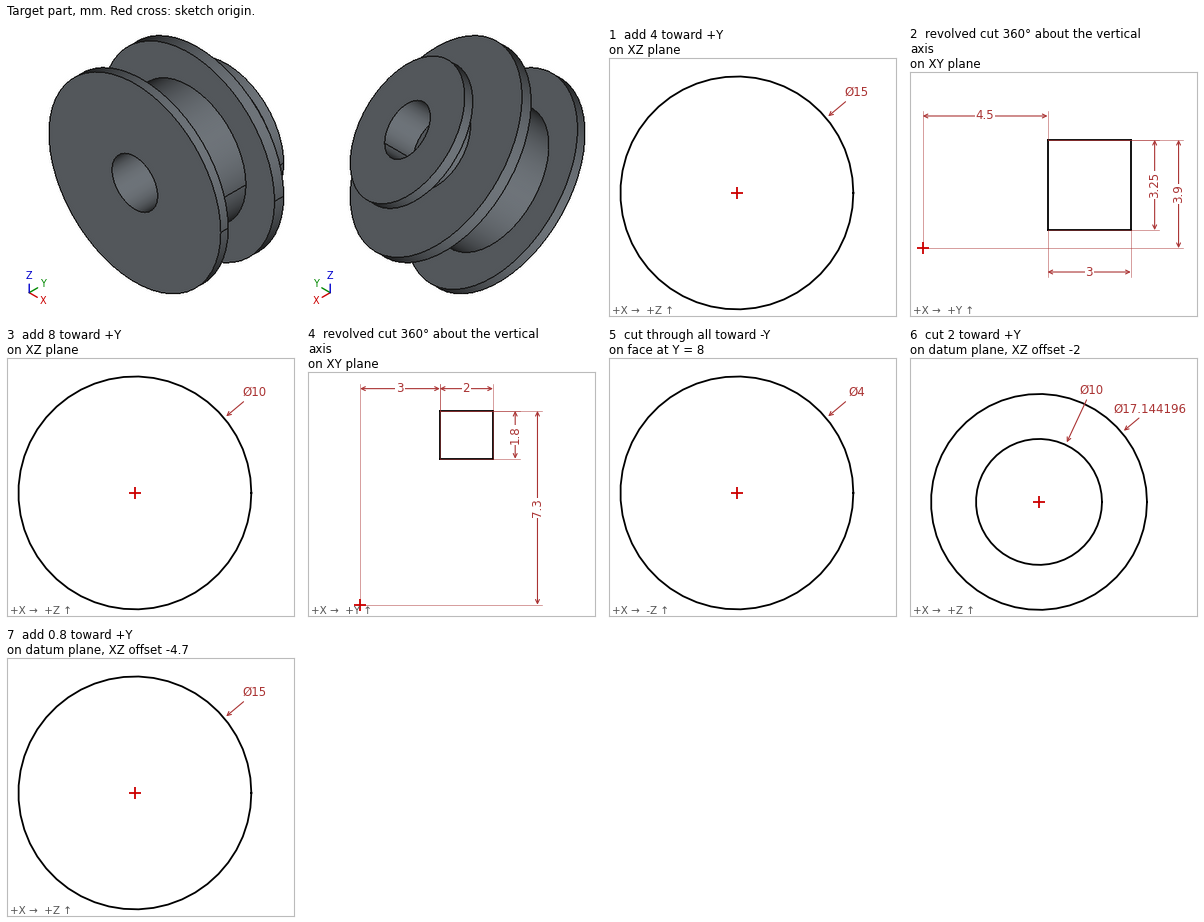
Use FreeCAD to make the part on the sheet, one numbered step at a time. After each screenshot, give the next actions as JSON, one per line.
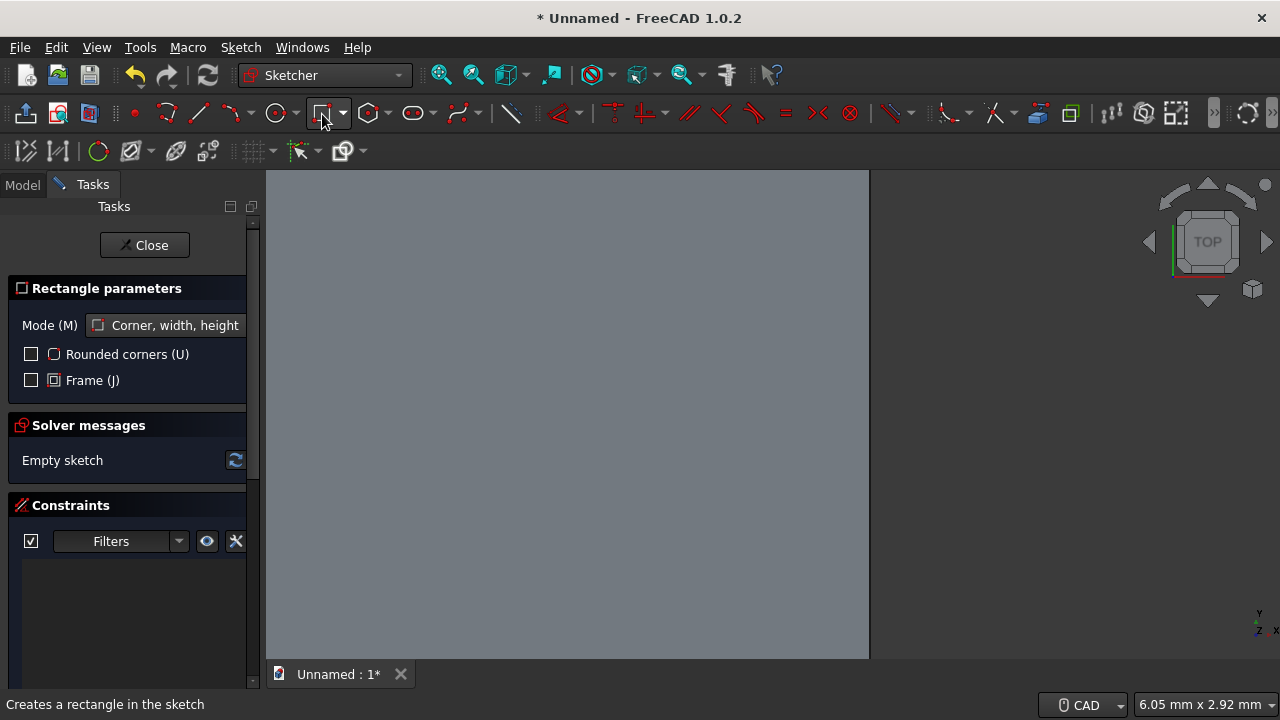
{"action": "left_click", "coordinate": [535, 259]}
{"action": "left_click", "coordinate": [870, 561]}
{"action": "key", "text": "Escape"}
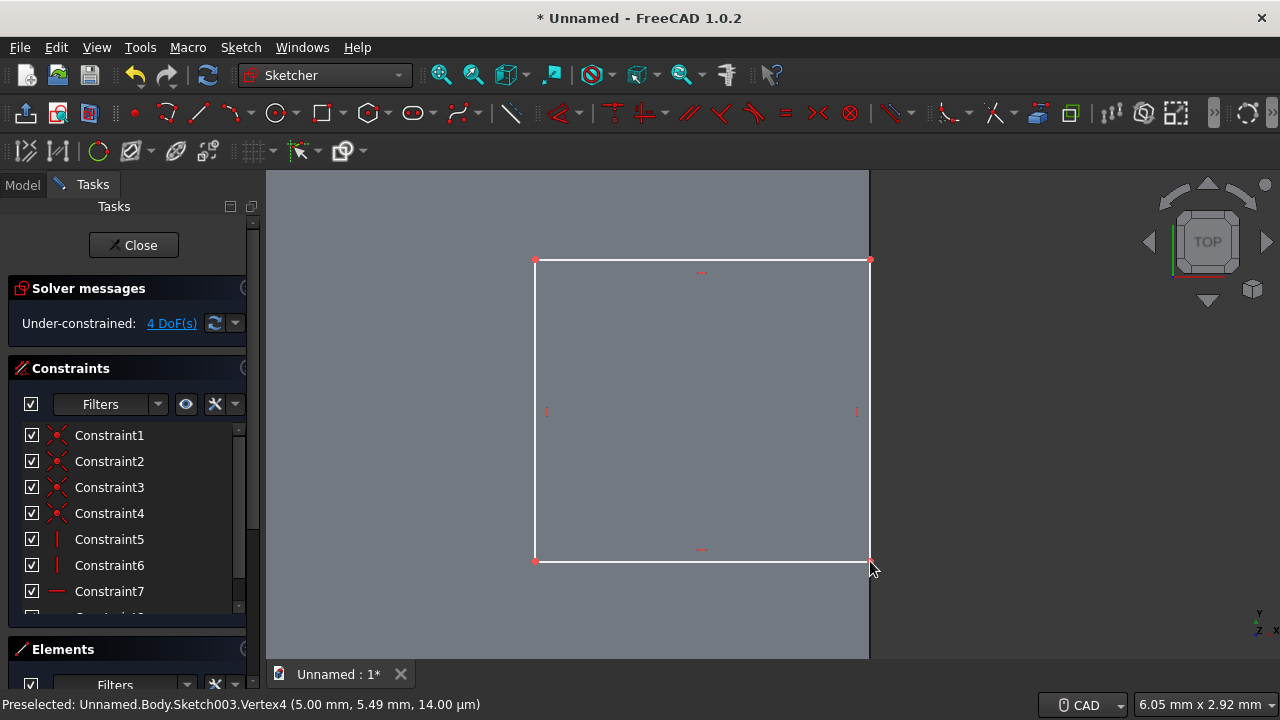
{"action": "left_click", "coordinate": [558, 114]}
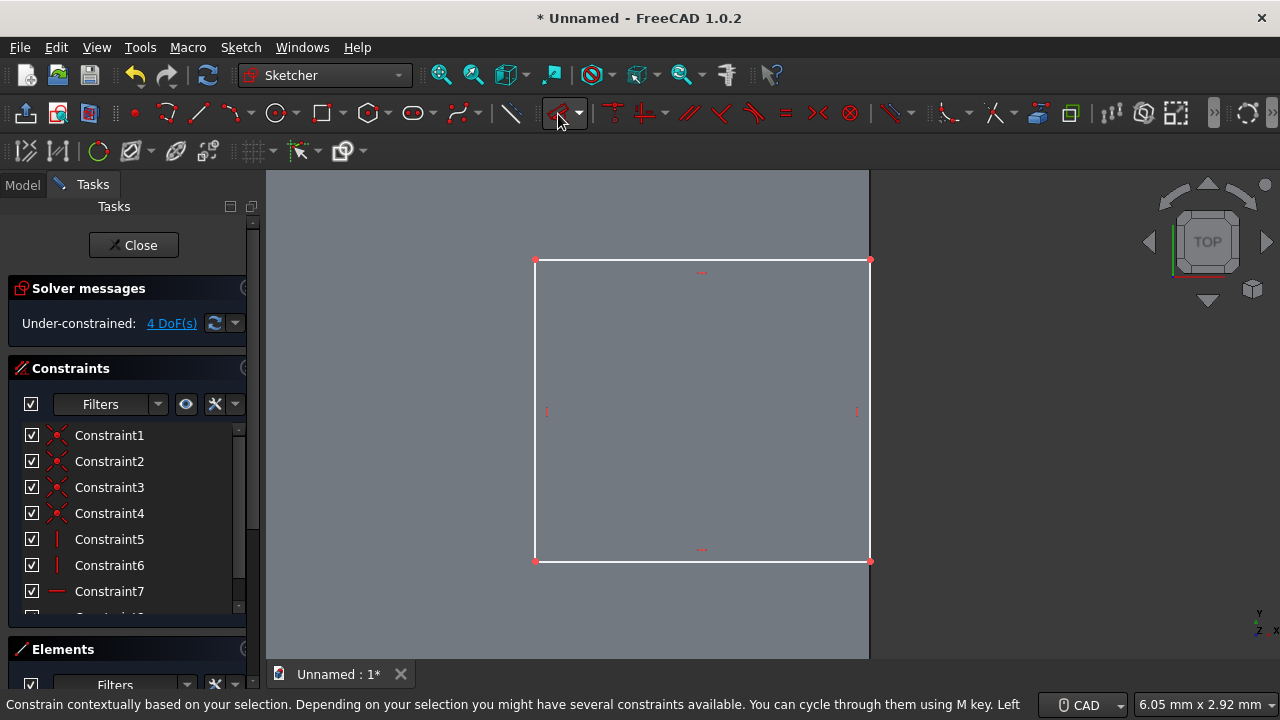
{"action": "left_click", "coordinate": [636, 562]}
{"action": "left_click", "coordinate": [703, 596]}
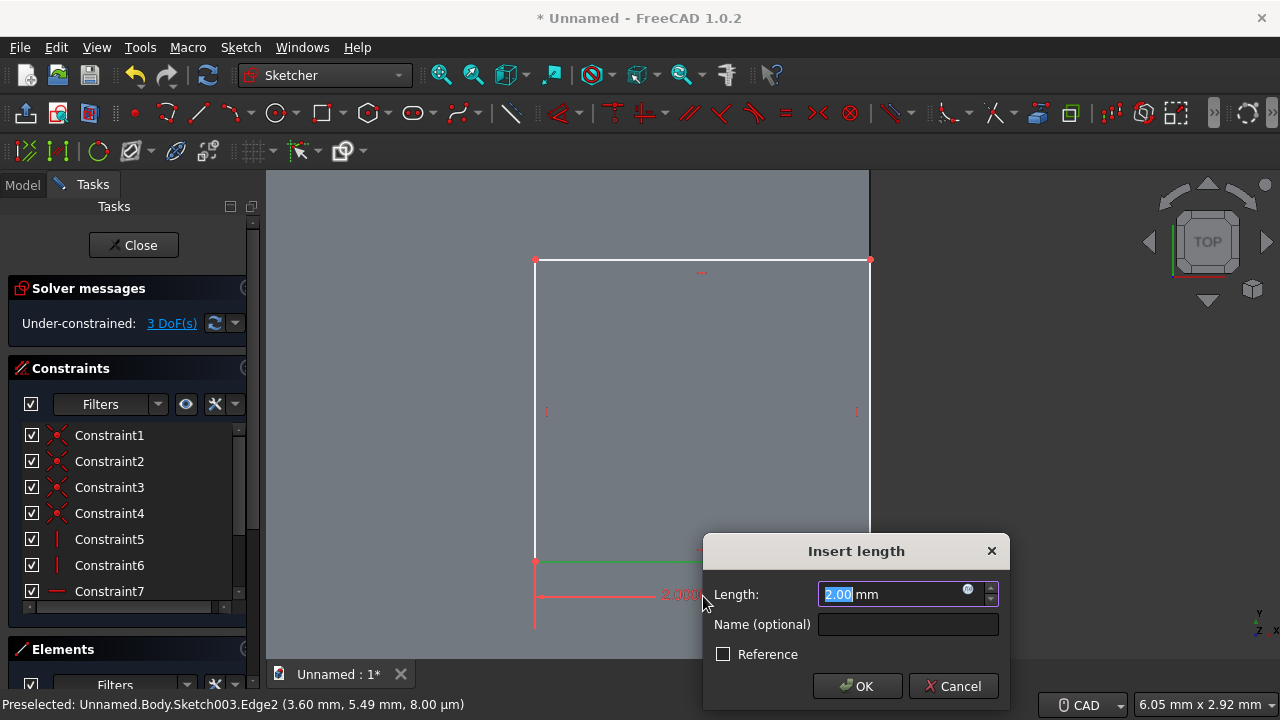
{"action": "type", "text": "2"}
{"action": "key", "text": "Return"}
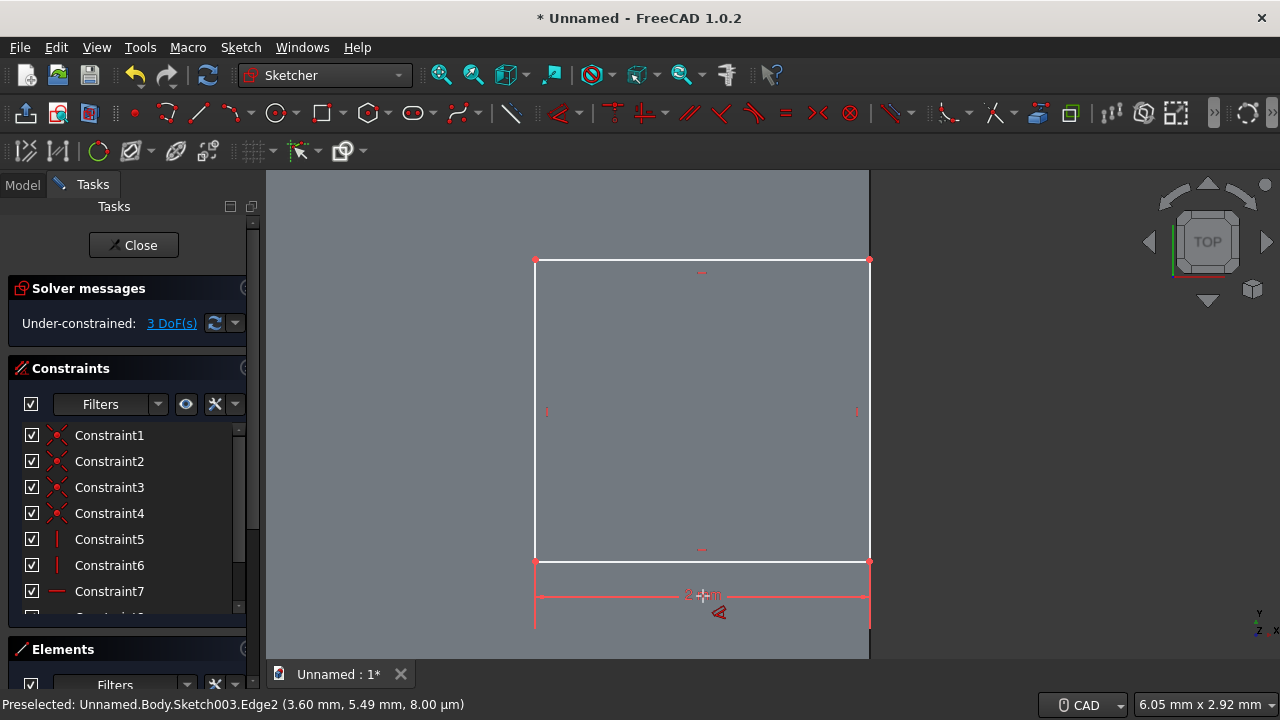
{"action": "left_click", "coordinate": [535, 260]}
{"action": "left_click", "coordinate": [415, 226]}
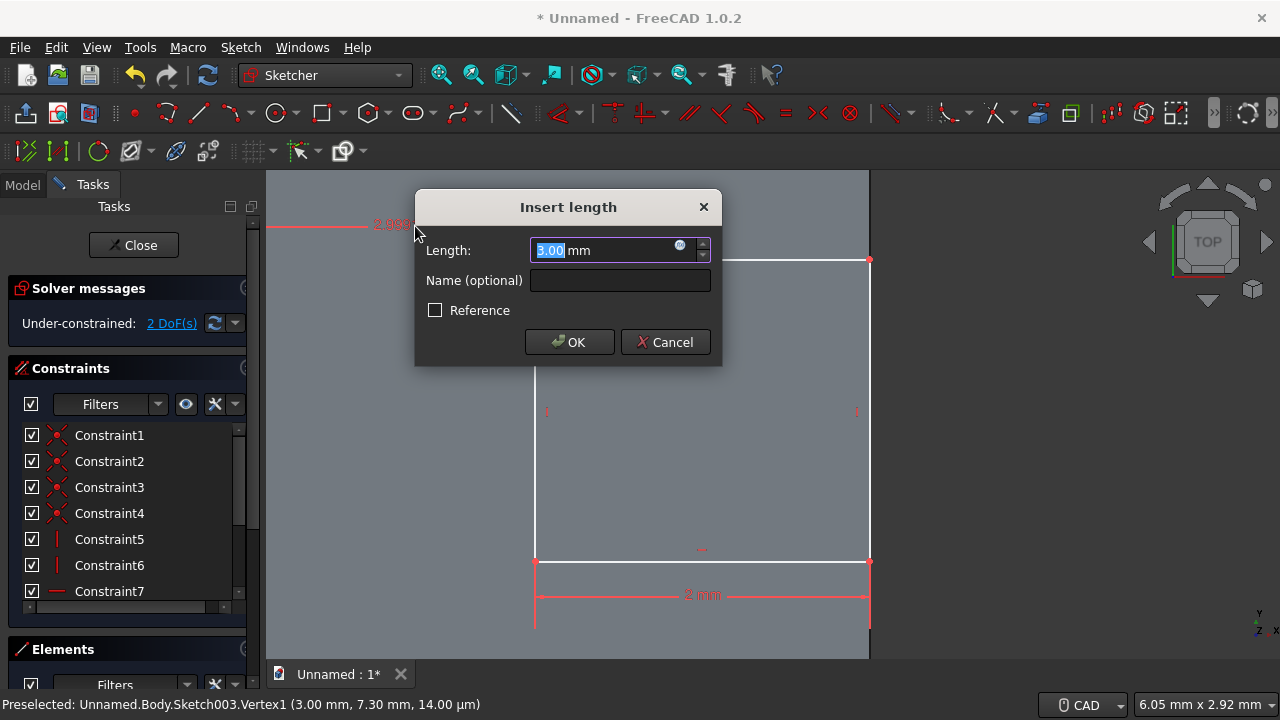
{"action": "type", "text": "3"}
{"action": "key", "text": "Return"}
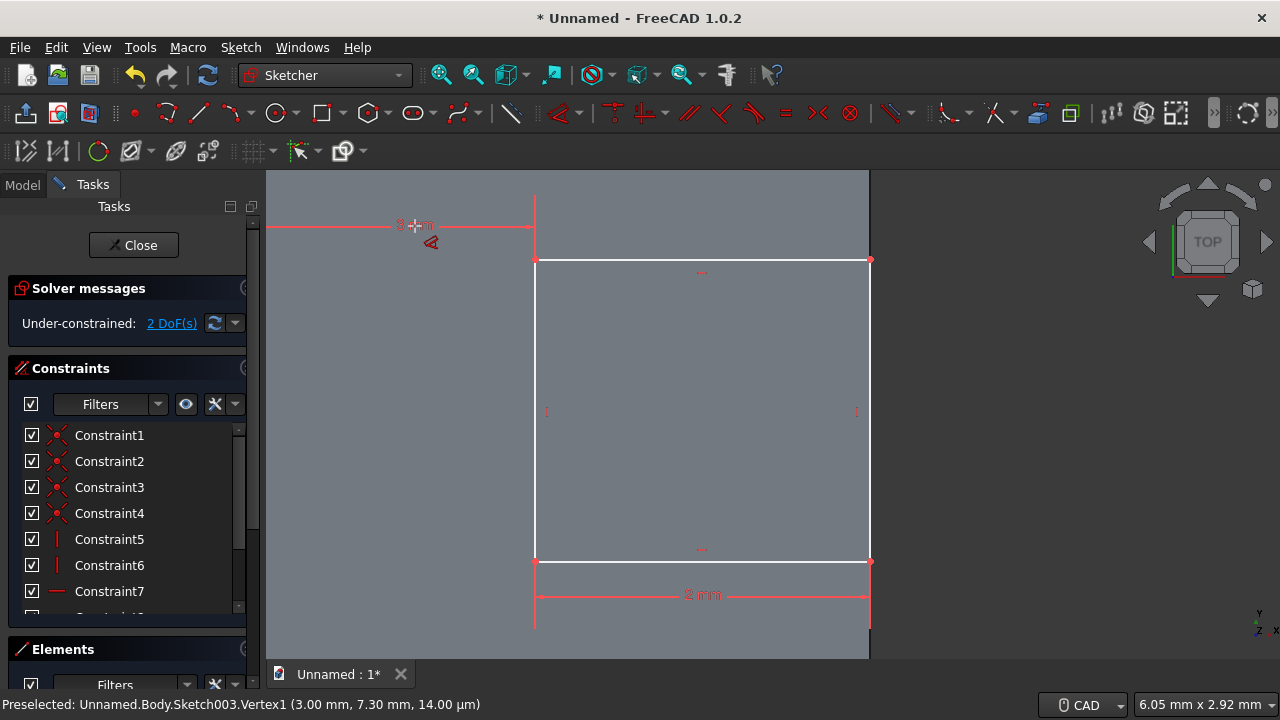
{"action": "left_click", "coordinate": [535, 351]}
{"action": "left_click", "coordinate": [501, 411]}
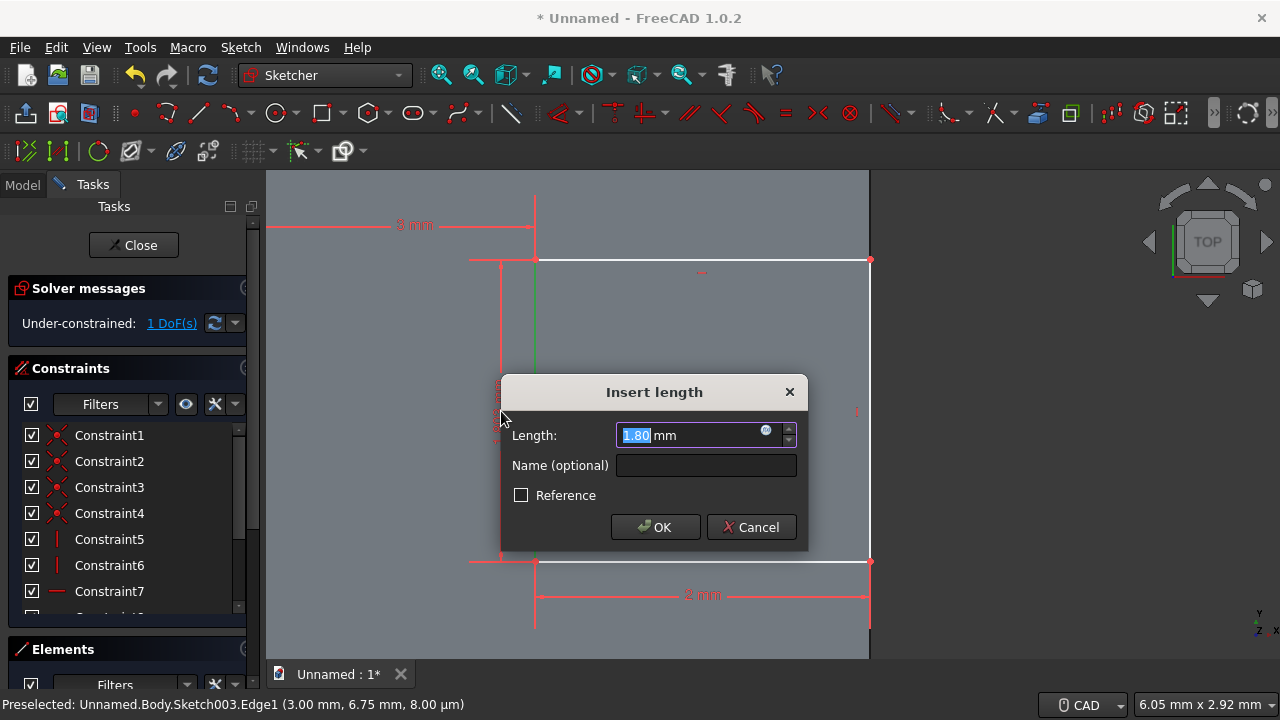
{"action": "type", "text": "1.8"}
{"action": "key", "text": "Return"}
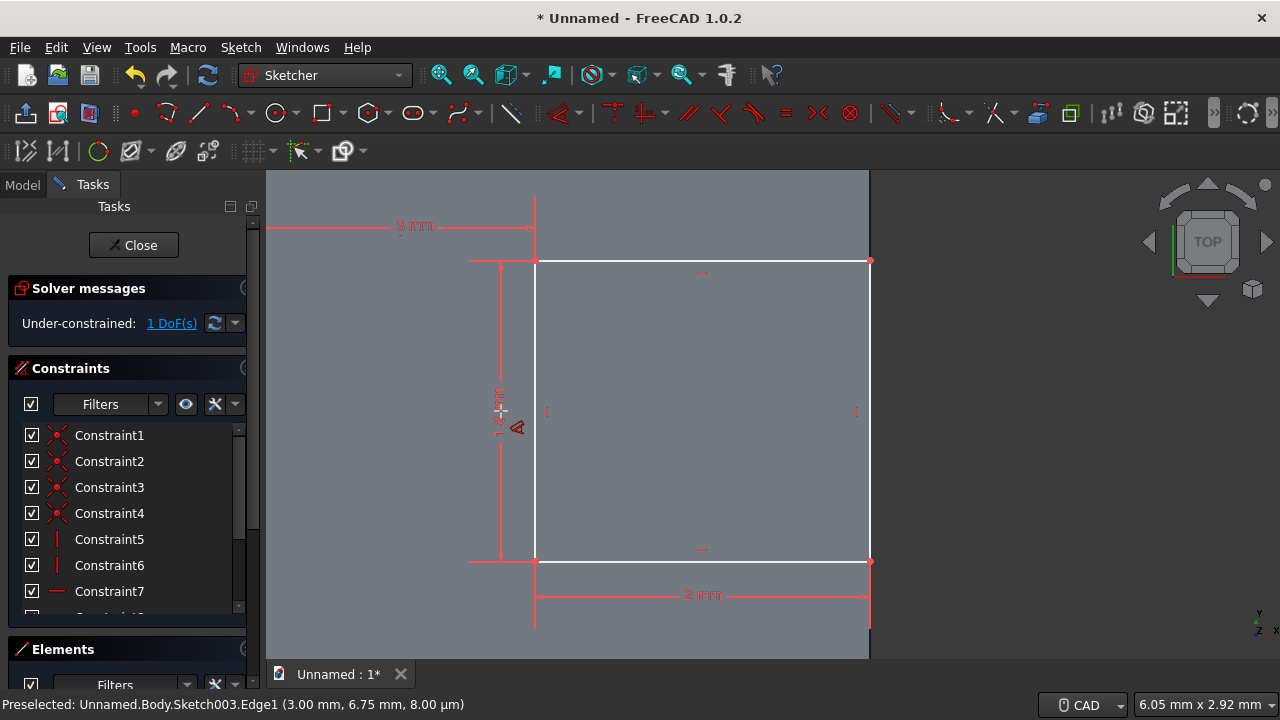
{"action": "left_click", "coordinate": [535, 261]}
{"action": "left_click", "coordinate": [569, 446]}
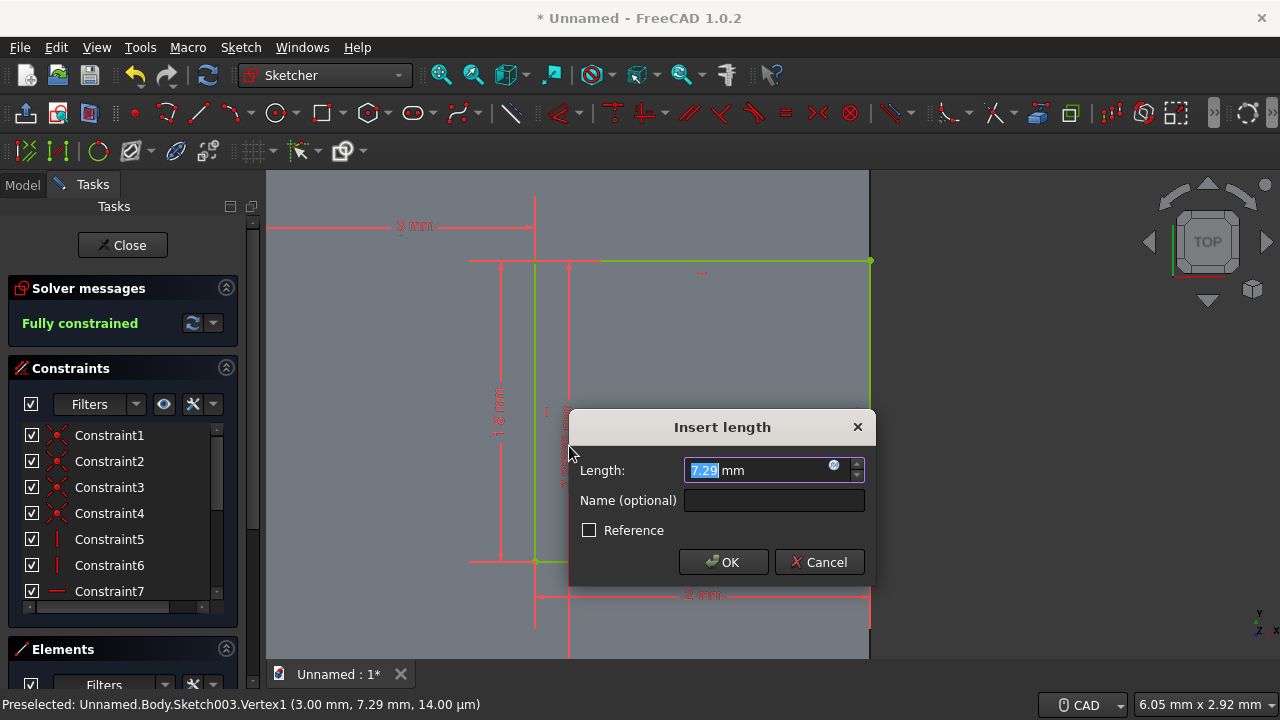
{"action": "type", "text": "7.3"}
{"action": "key", "text": "Return"}
{"action": "key", "text": "Escape"}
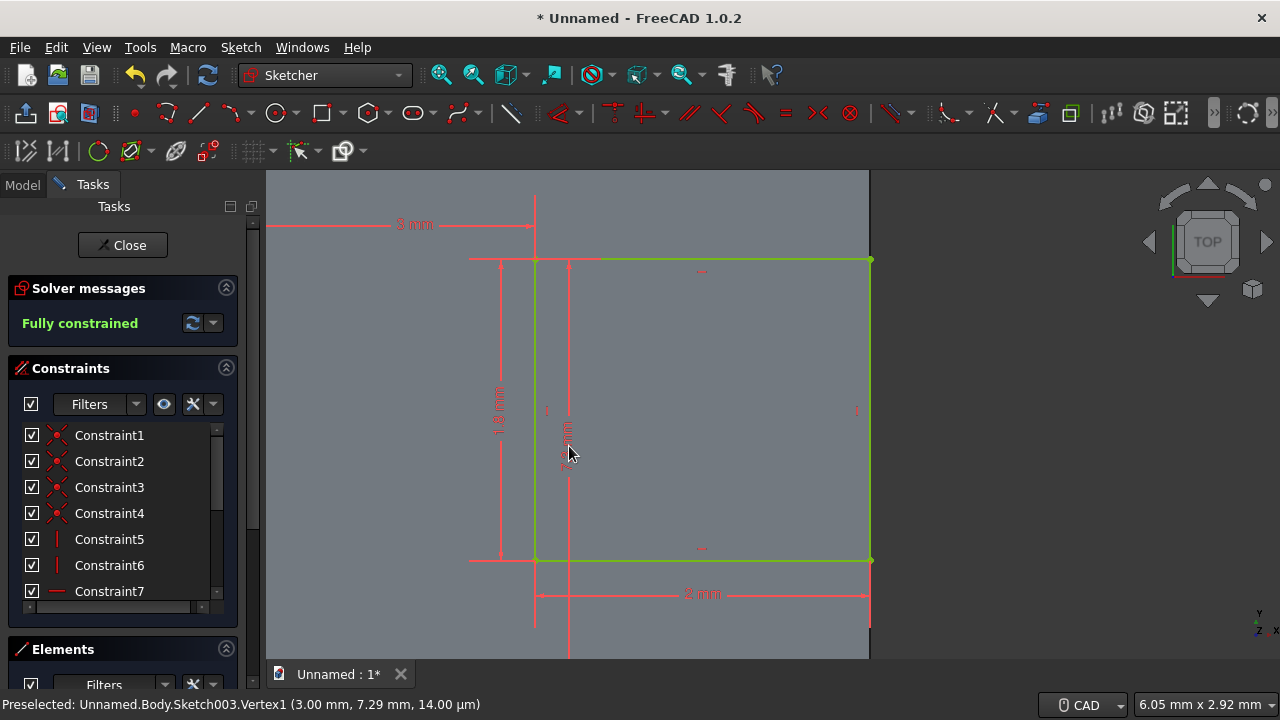
{"action": "left_click", "coordinate": [123, 245]}